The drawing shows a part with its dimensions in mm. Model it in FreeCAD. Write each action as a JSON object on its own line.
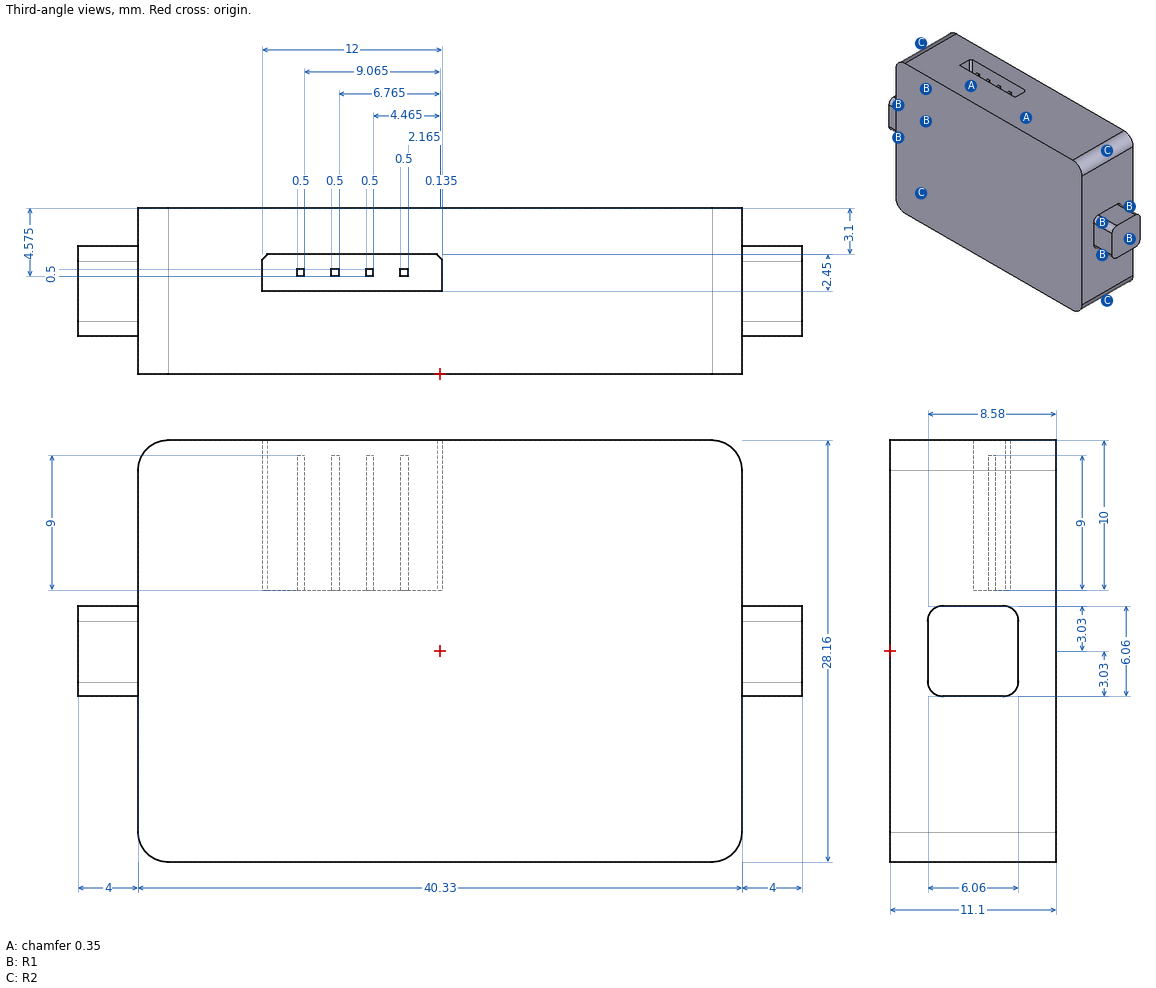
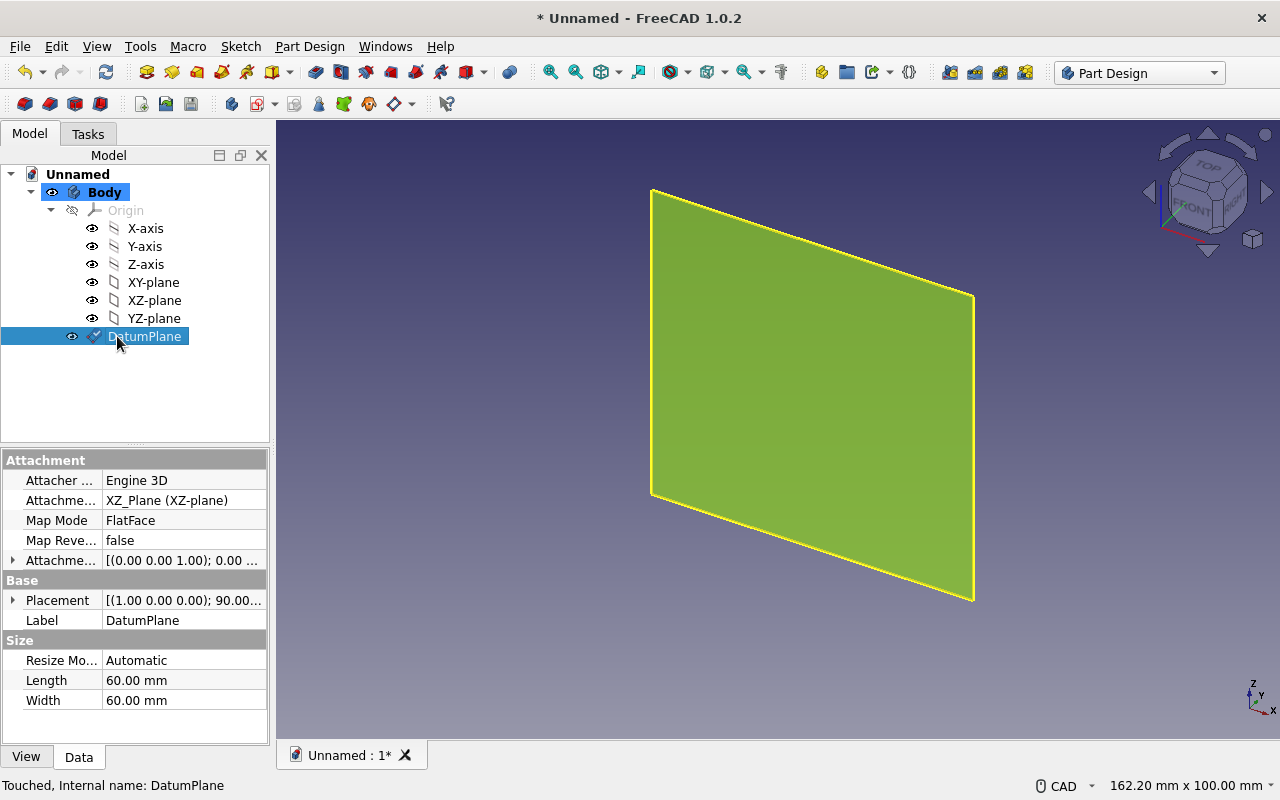
{"action": "left_click", "coordinate": [256, 104]}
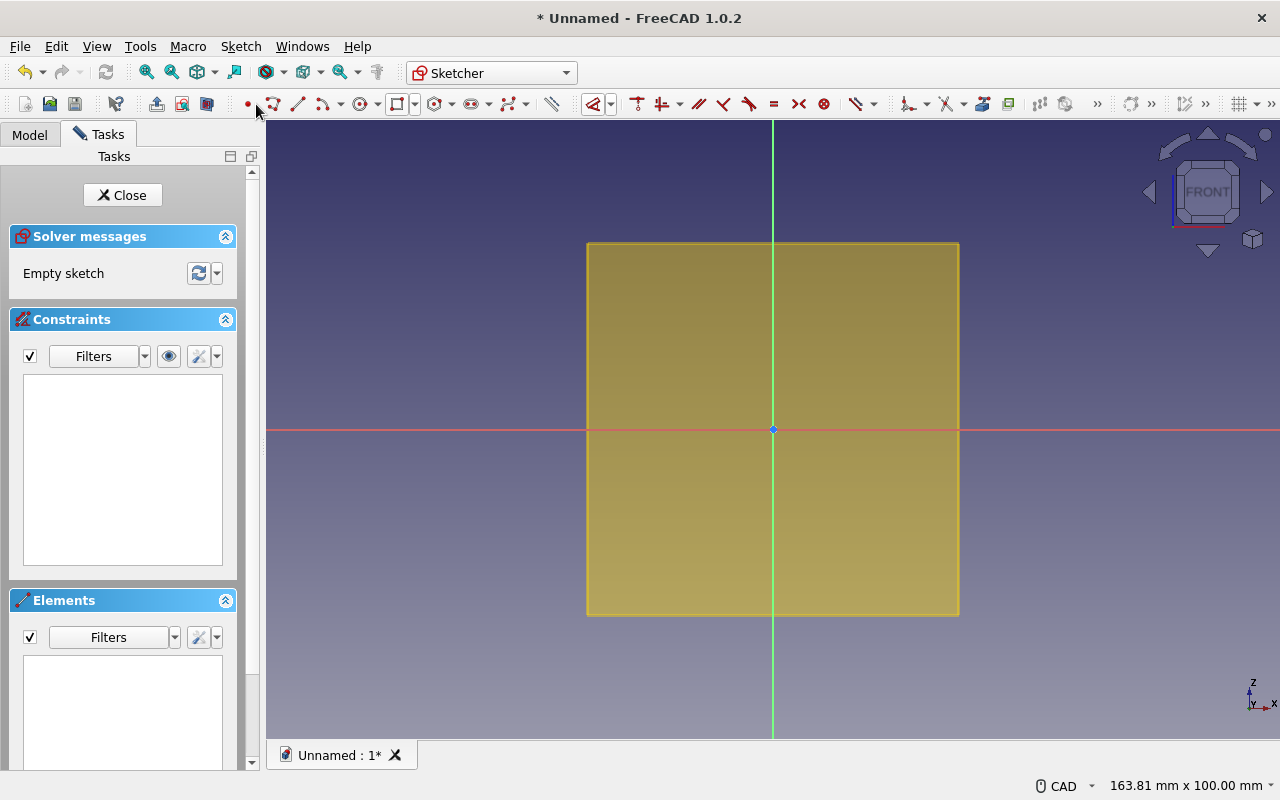
{"action": "scroll", "coordinate": [829, 430], "scroll_direction": "up", "scroll_amount": 4}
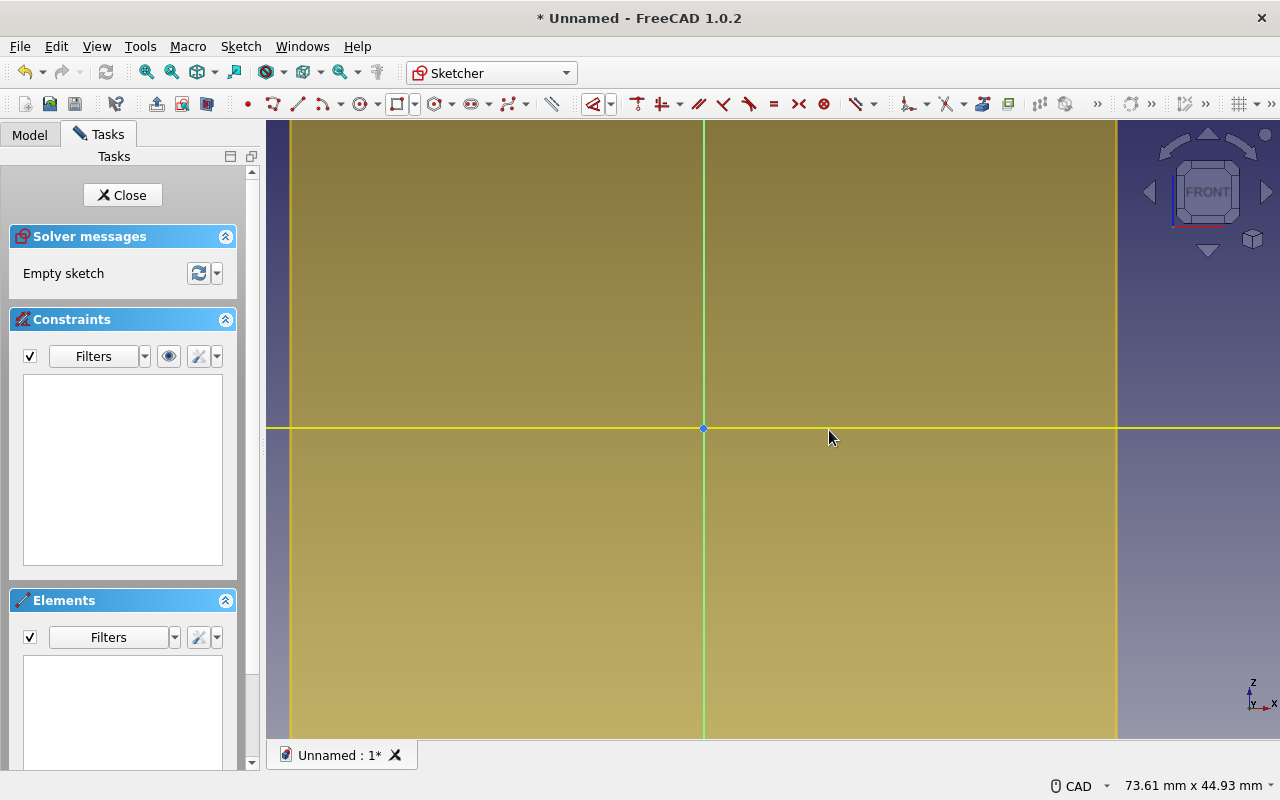
{"action": "key", "text": "g v"}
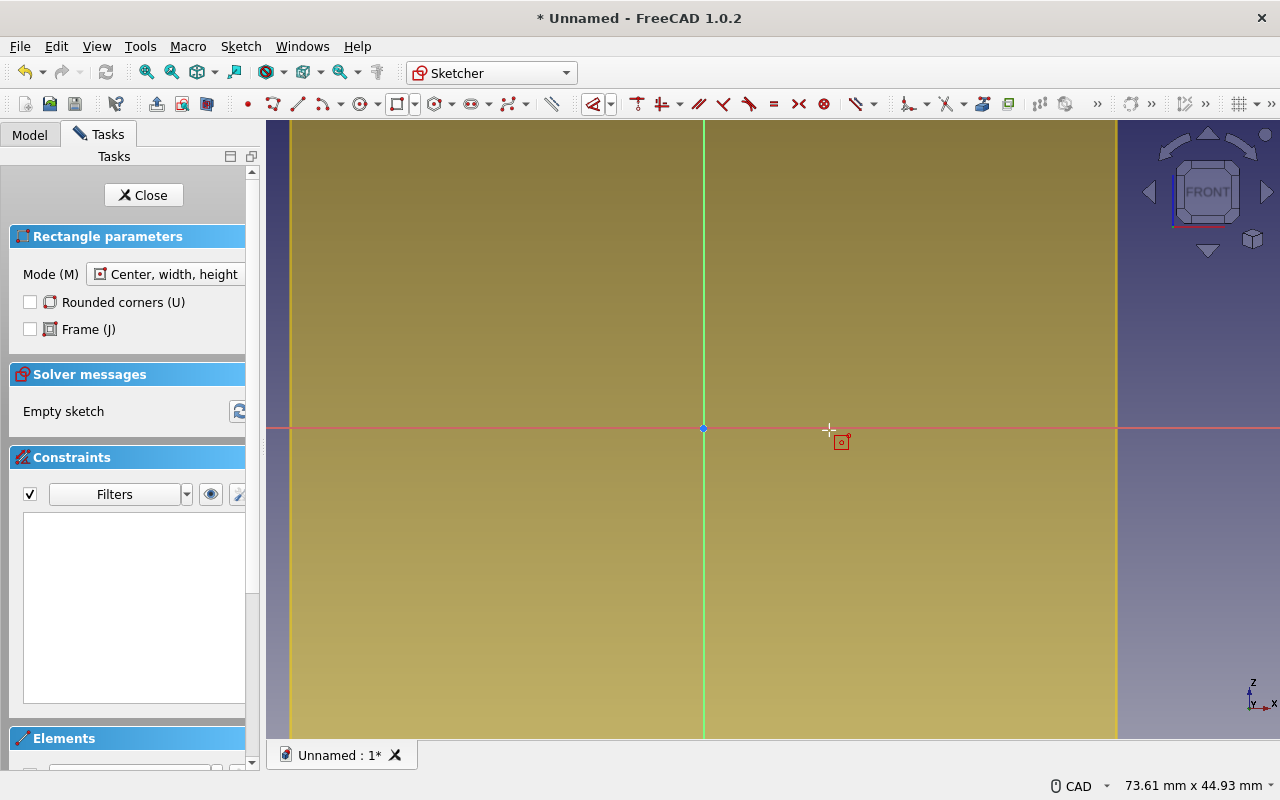
{"action": "left_click", "coordinate": [704, 428]}
{"action": "mouse_move", "coordinate": [981, 234]}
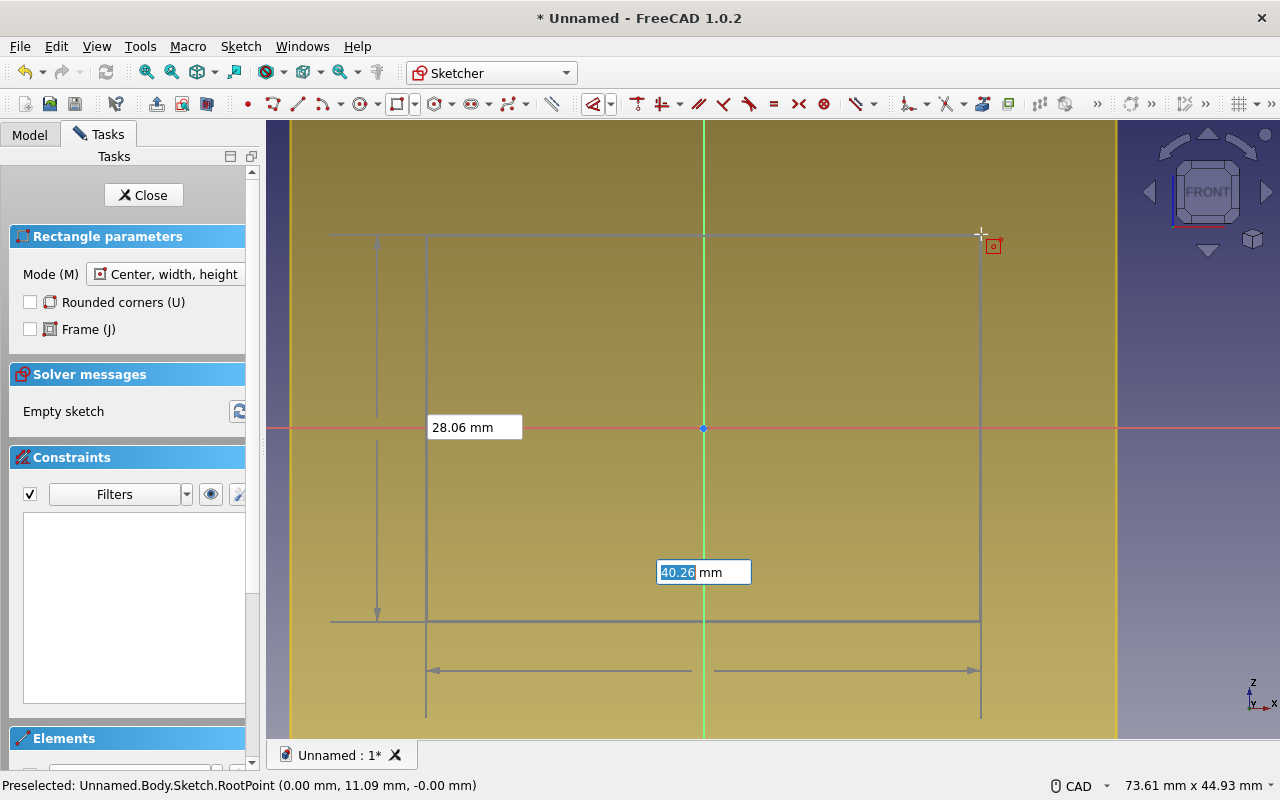
{"action": "type", "text": "40.33"}
{"action": "key", "text": "Tab"}
{"action": "type", "text": "28.16"}
{"action": "key", "text": "Return"}
{"action": "key", "text": "Escape"}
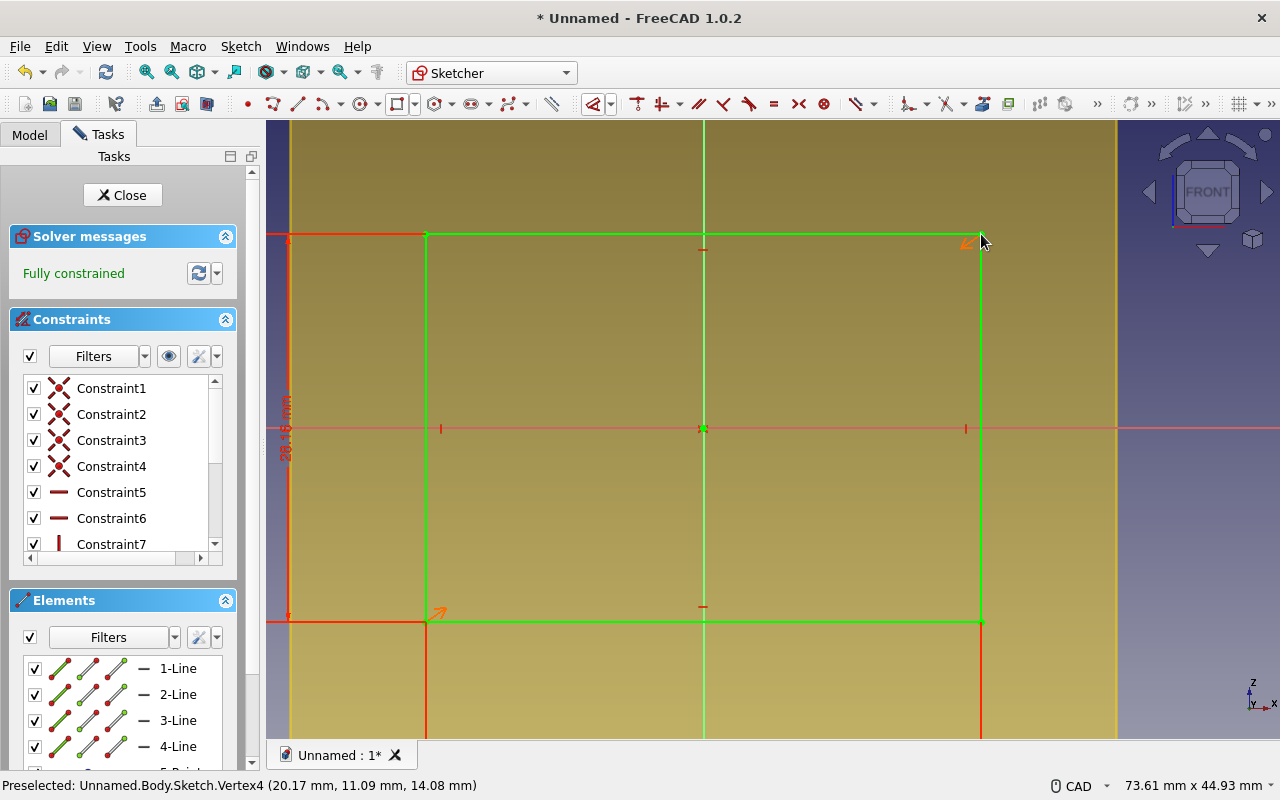
{"action": "left_click", "coordinate": [123, 195]}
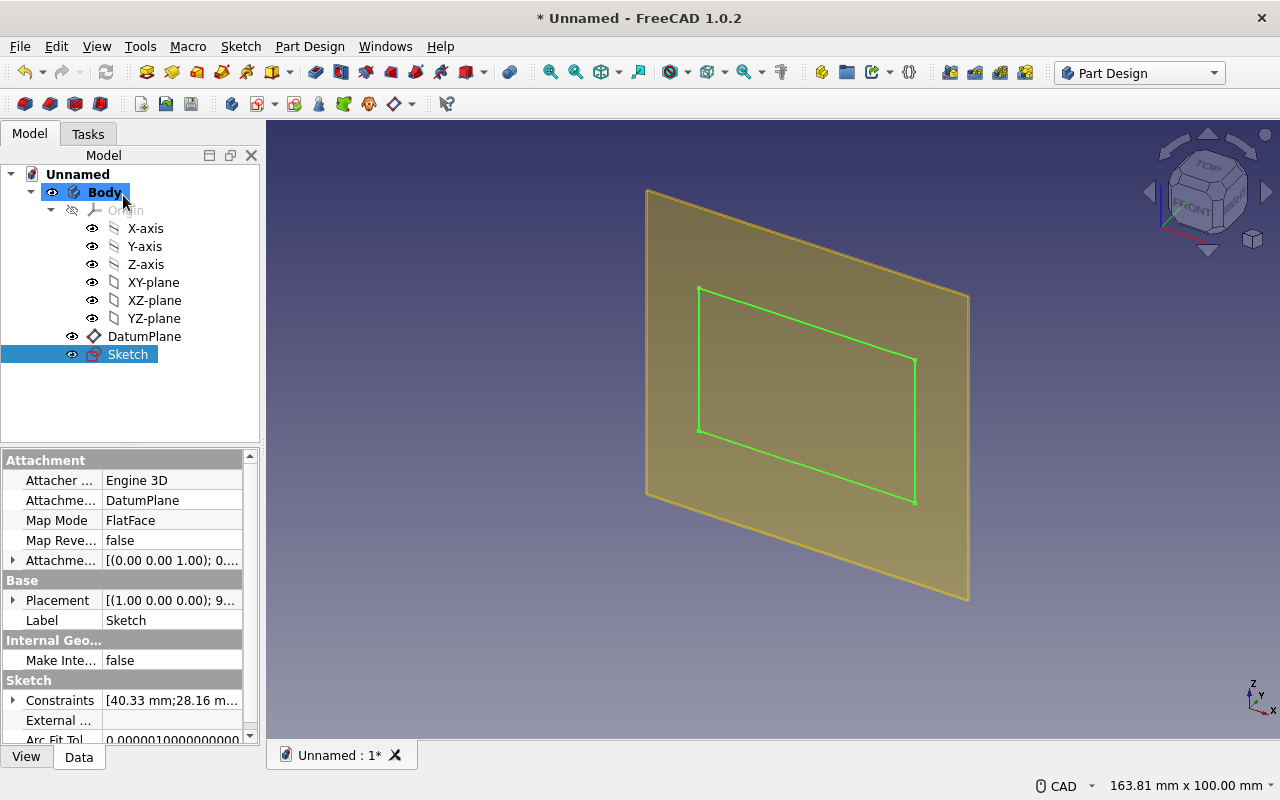
{"action": "left_click", "coordinate": [147, 72]}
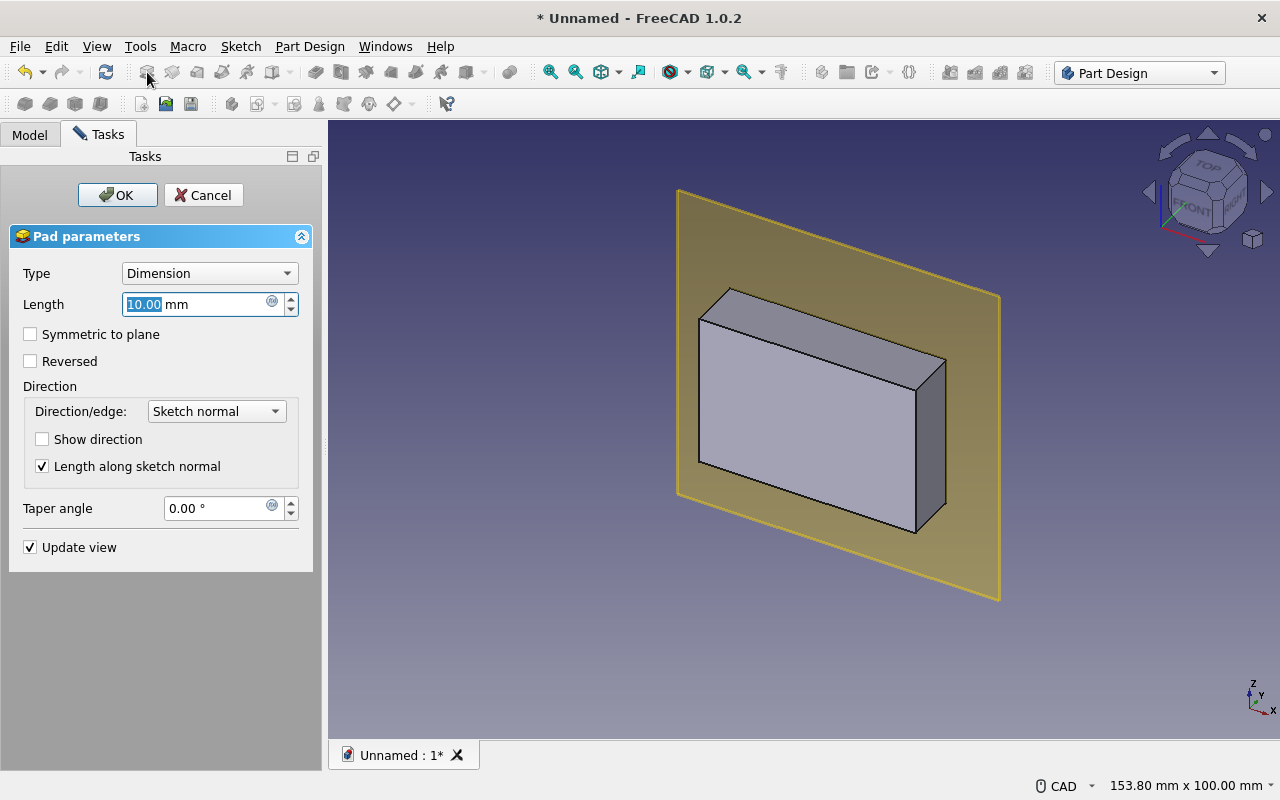
{"action": "type", "text": "11.1"}
{"action": "key", "text": "Tab"}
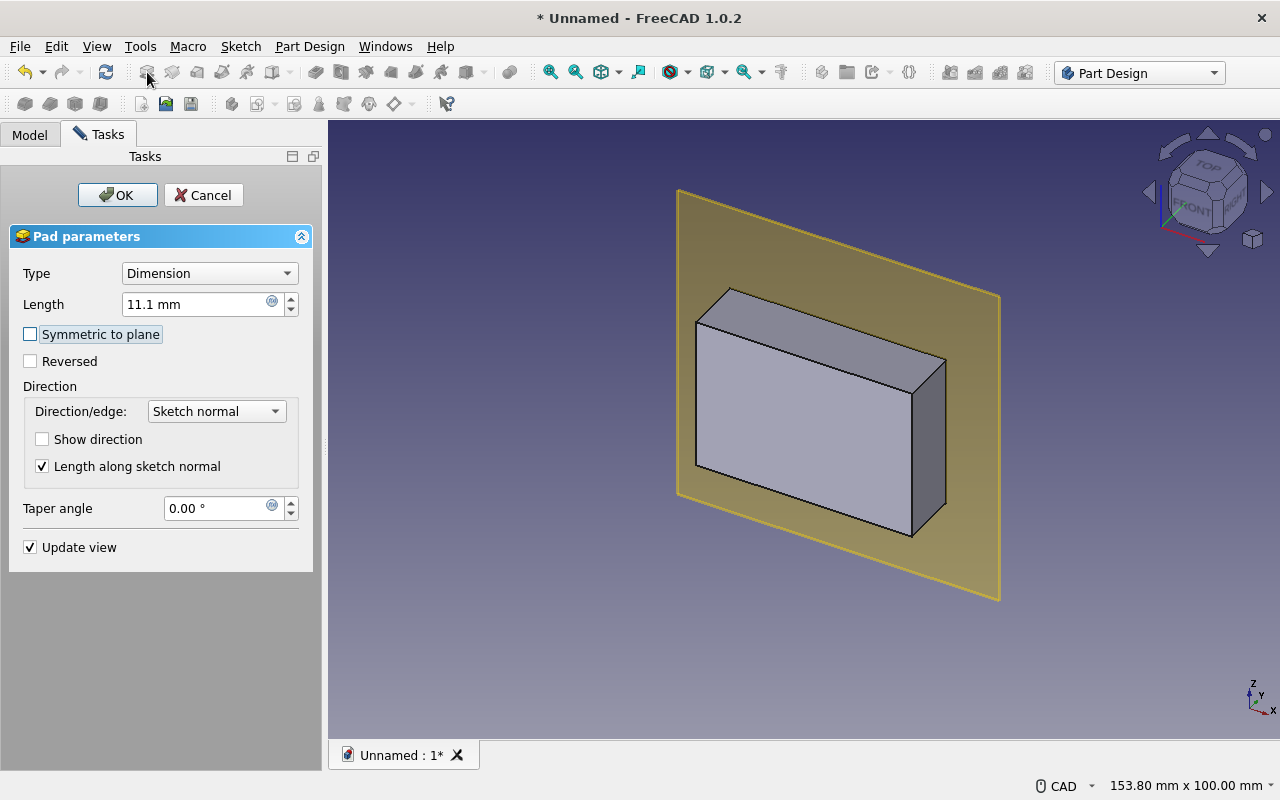
{"action": "left_click", "coordinate": [118, 195]}